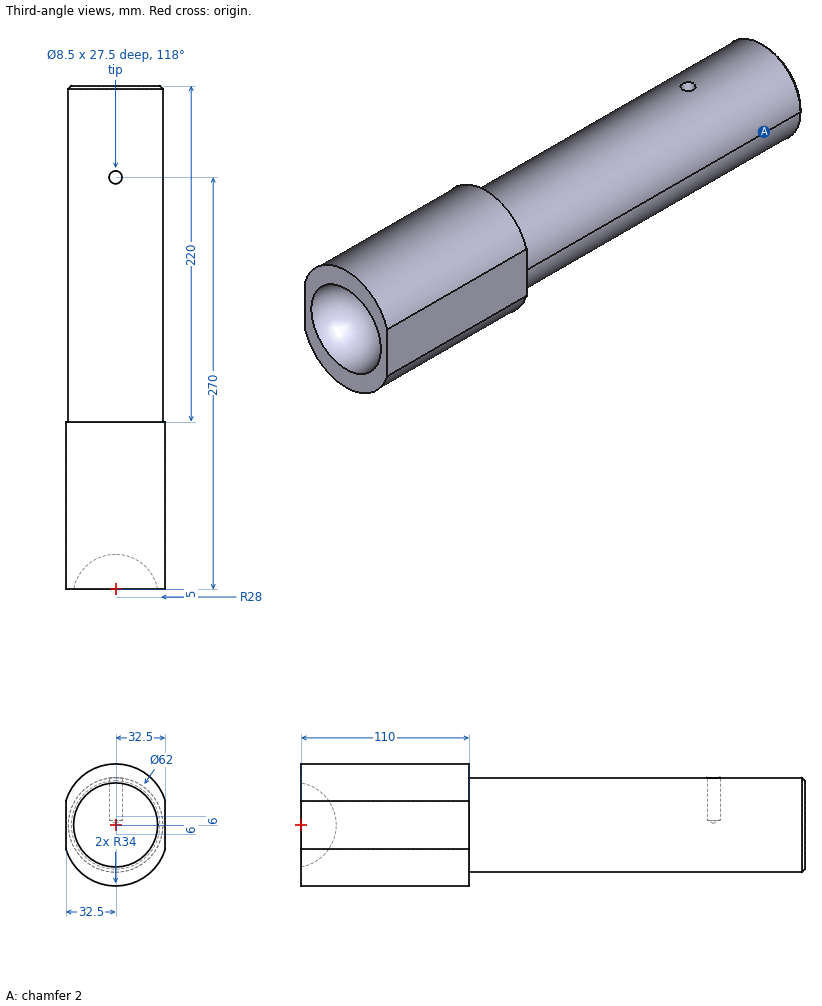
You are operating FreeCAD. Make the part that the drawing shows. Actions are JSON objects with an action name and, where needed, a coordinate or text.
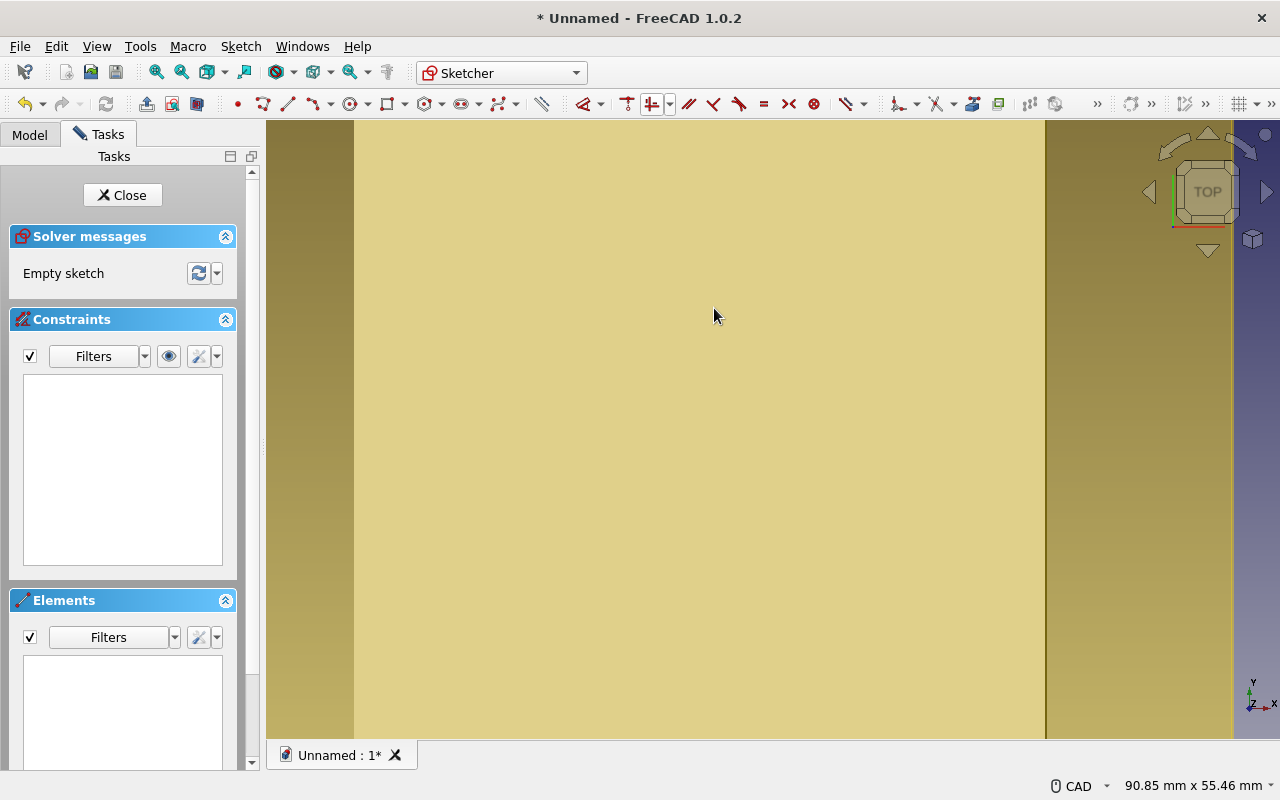
{"action": "scroll", "coordinate": [698, 412], "scroll_direction": "up", "scroll_amount": 7}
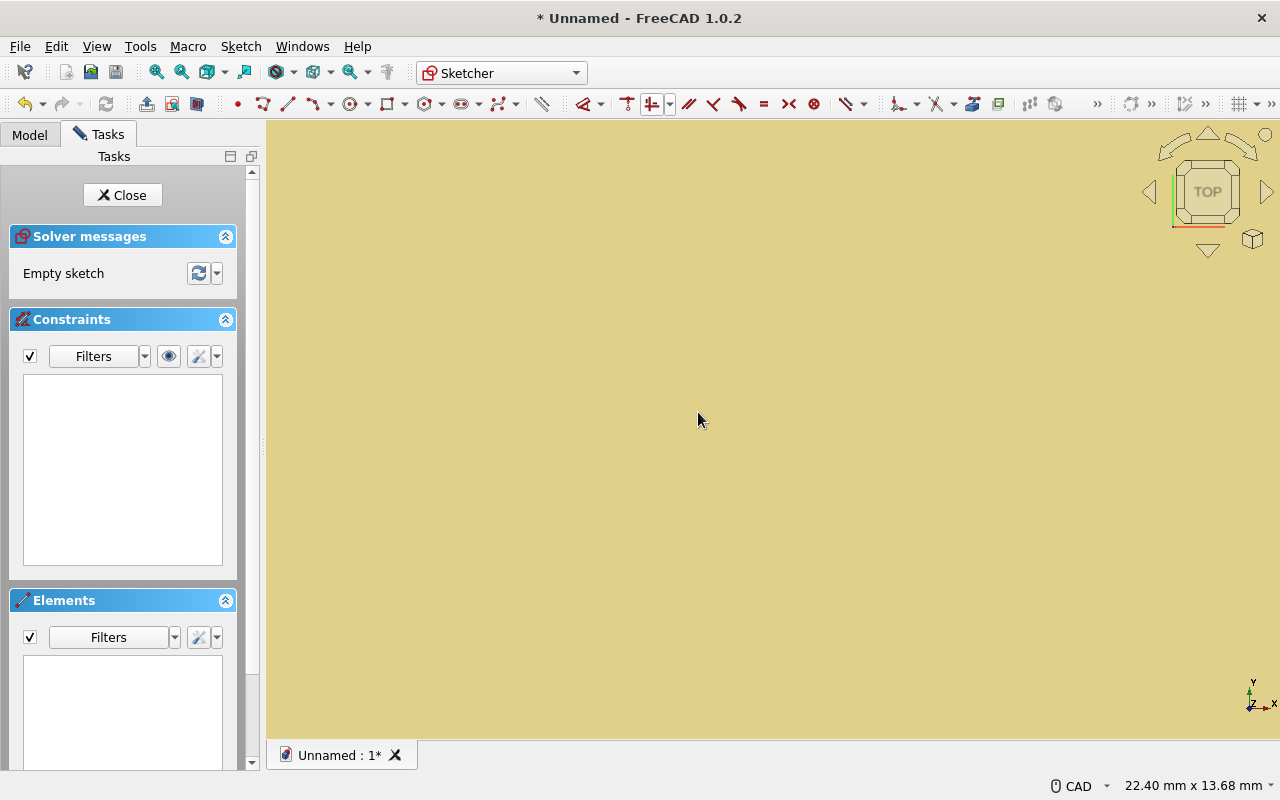
{"action": "key", "text": "g c"}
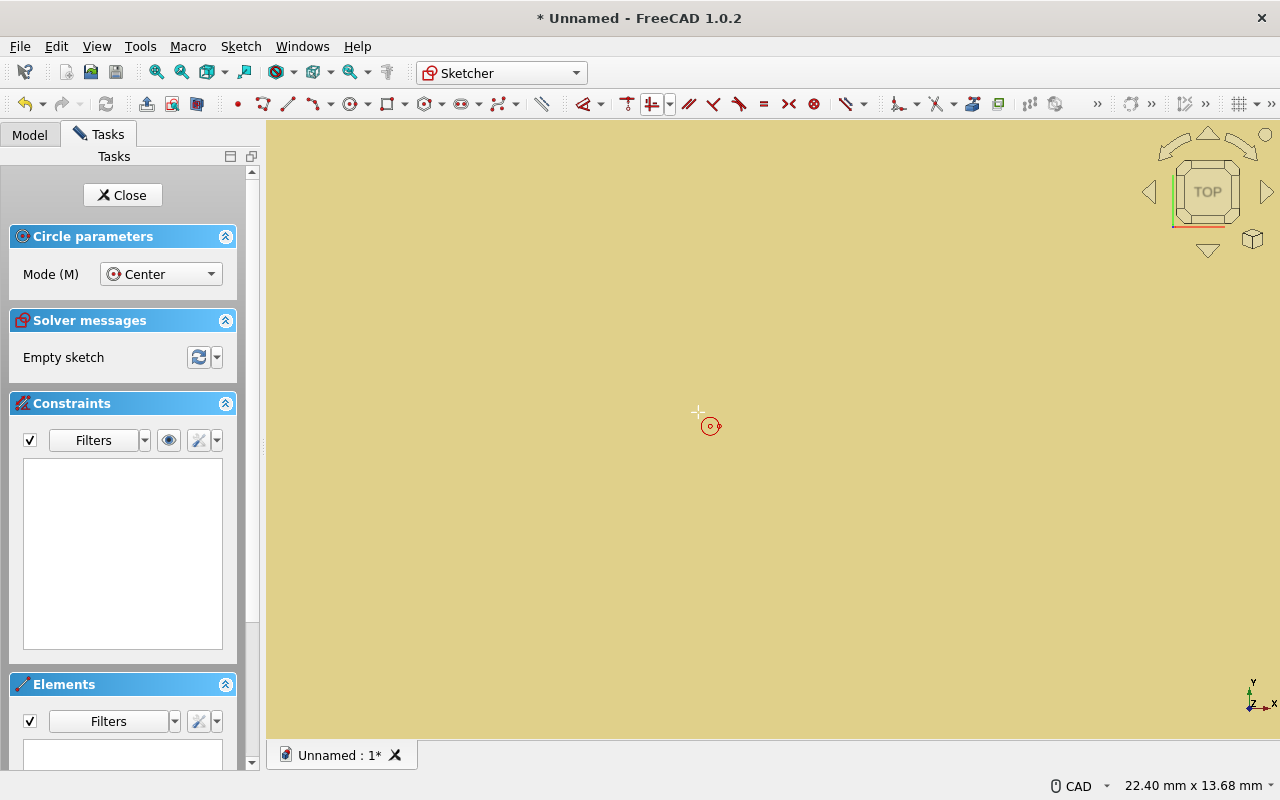
{"action": "left_click", "coordinate": [704, 427]}
{"action": "mouse_move", "coordinate": [840, 291]}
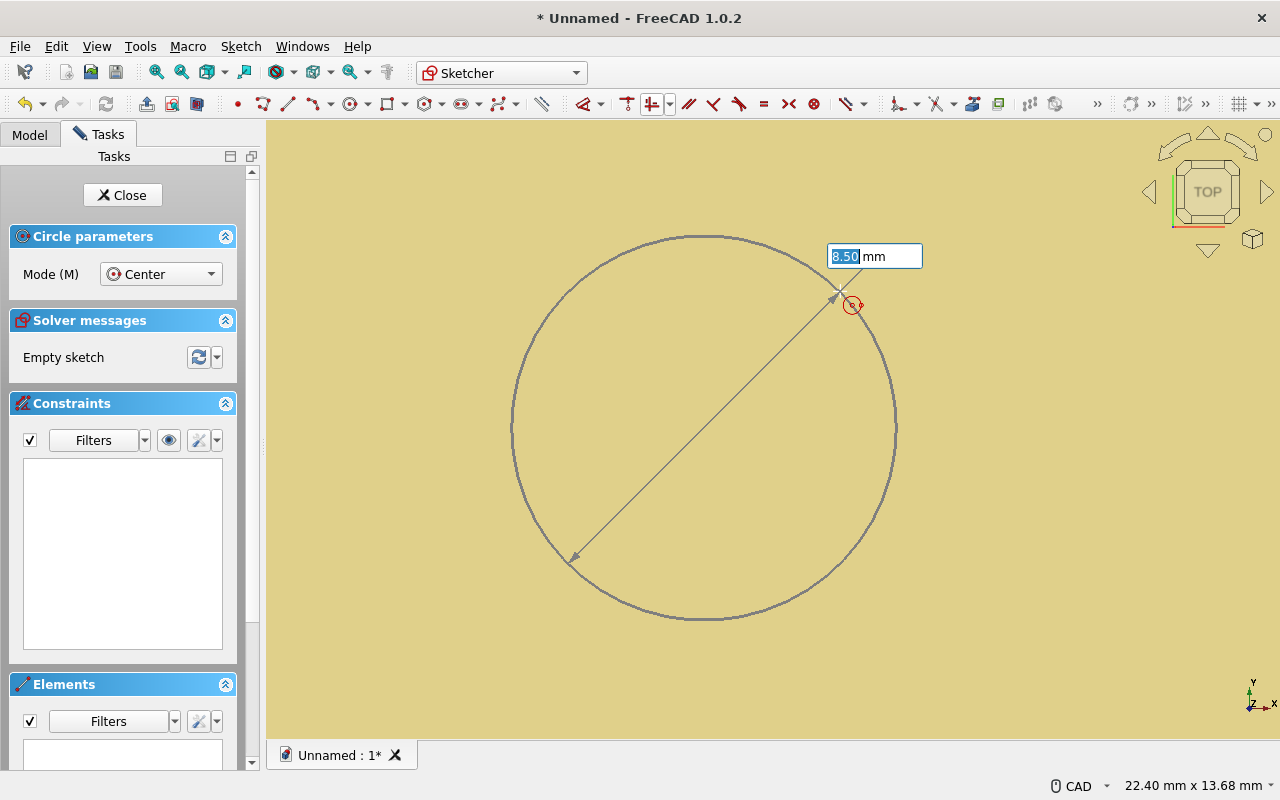
{"action": "type", "text": "8.5"}
{"action": "key", "text": "Return"}
{"action": "key", "text": "Escape"}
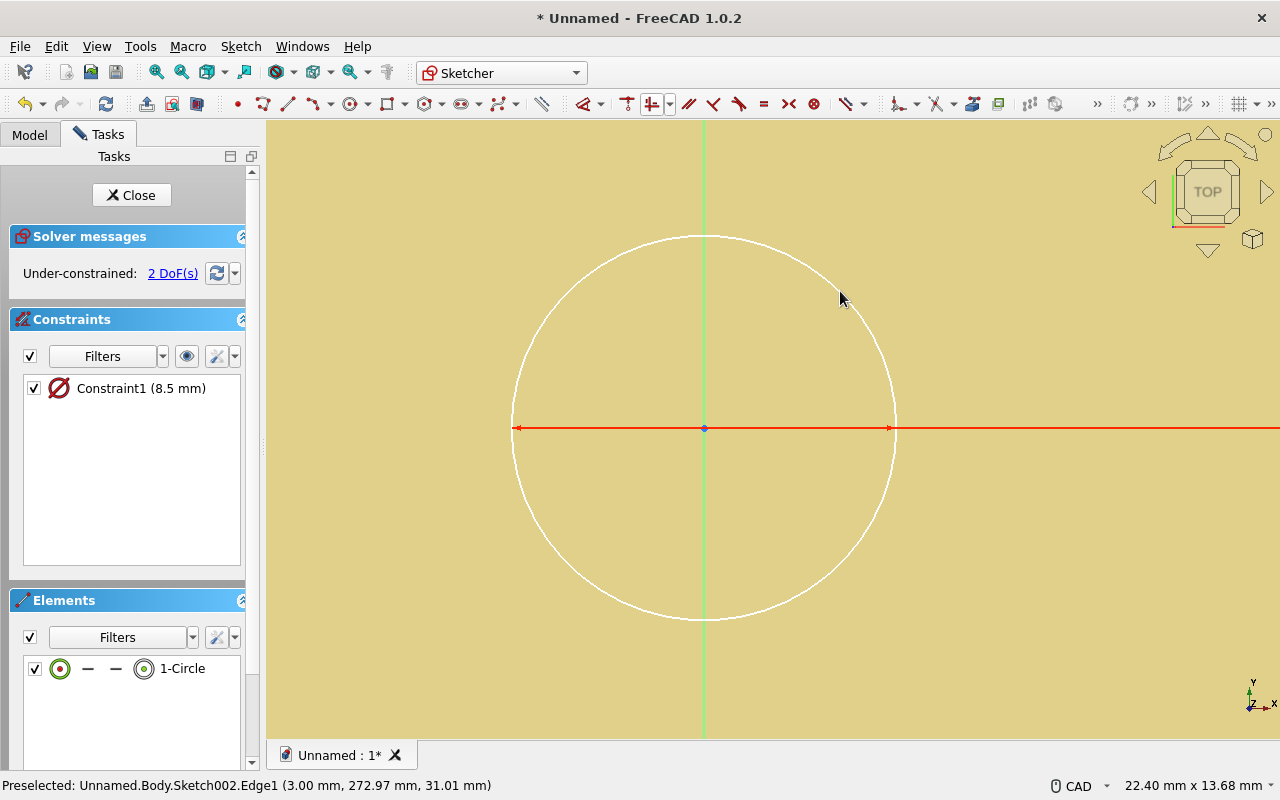
{"action": "left_click", "coordinate": [704, 428]}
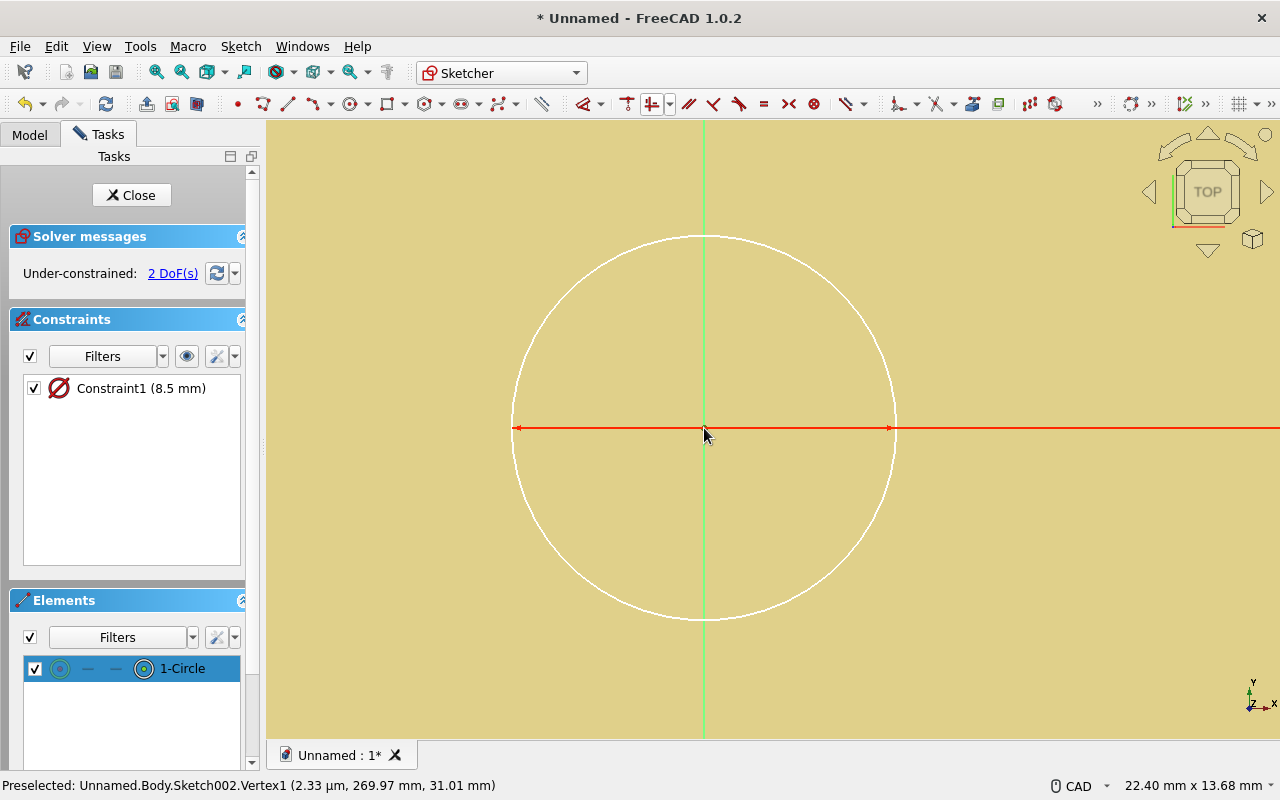
{"action": "left_click", "coordinate": [704, 671]}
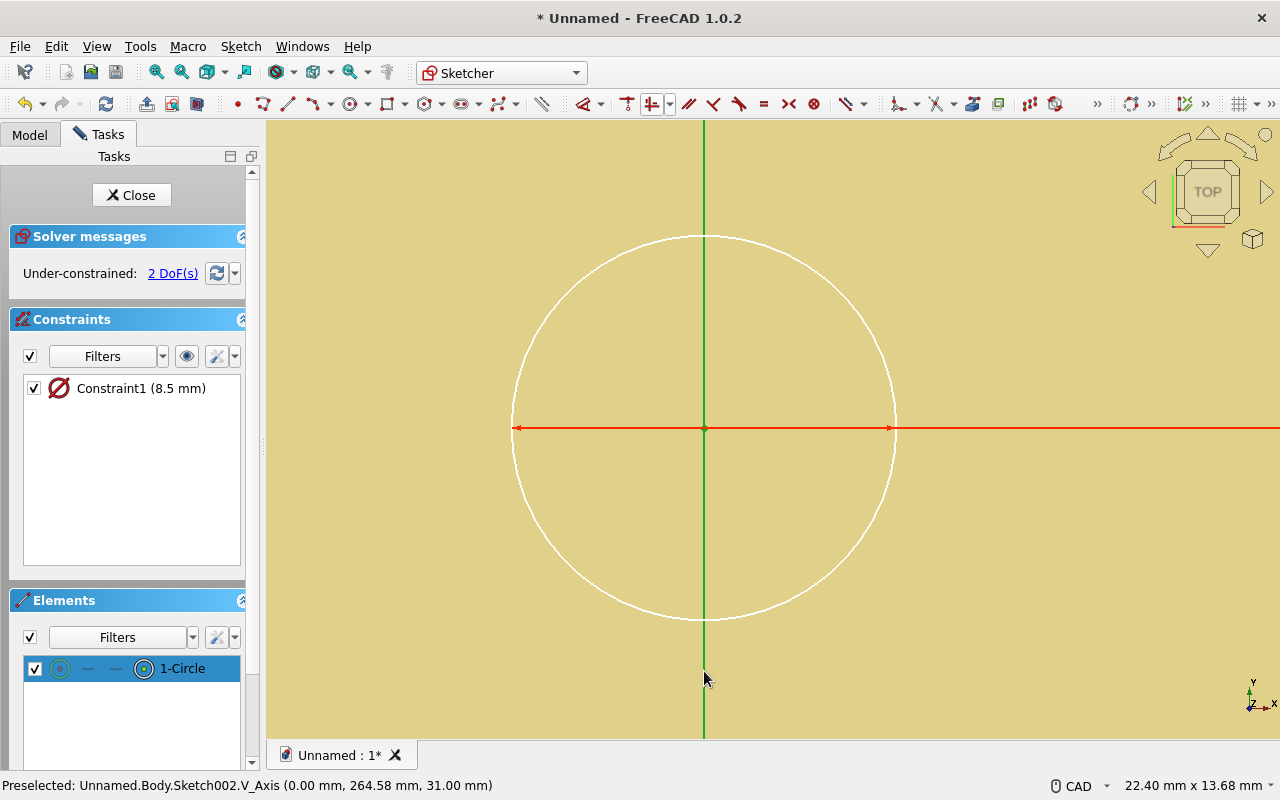
{"action": "left_click", "coordinate": [627, 104]}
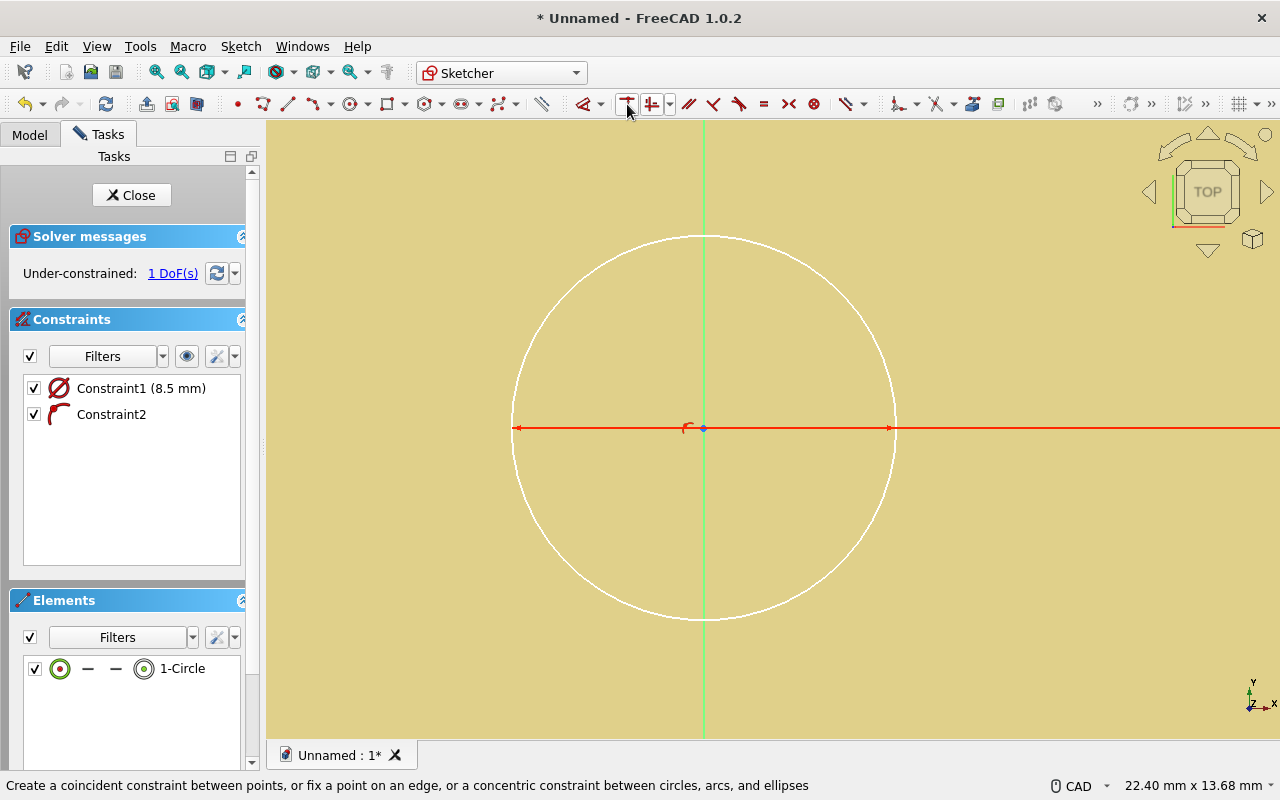
{"action": "key", "text": "d"}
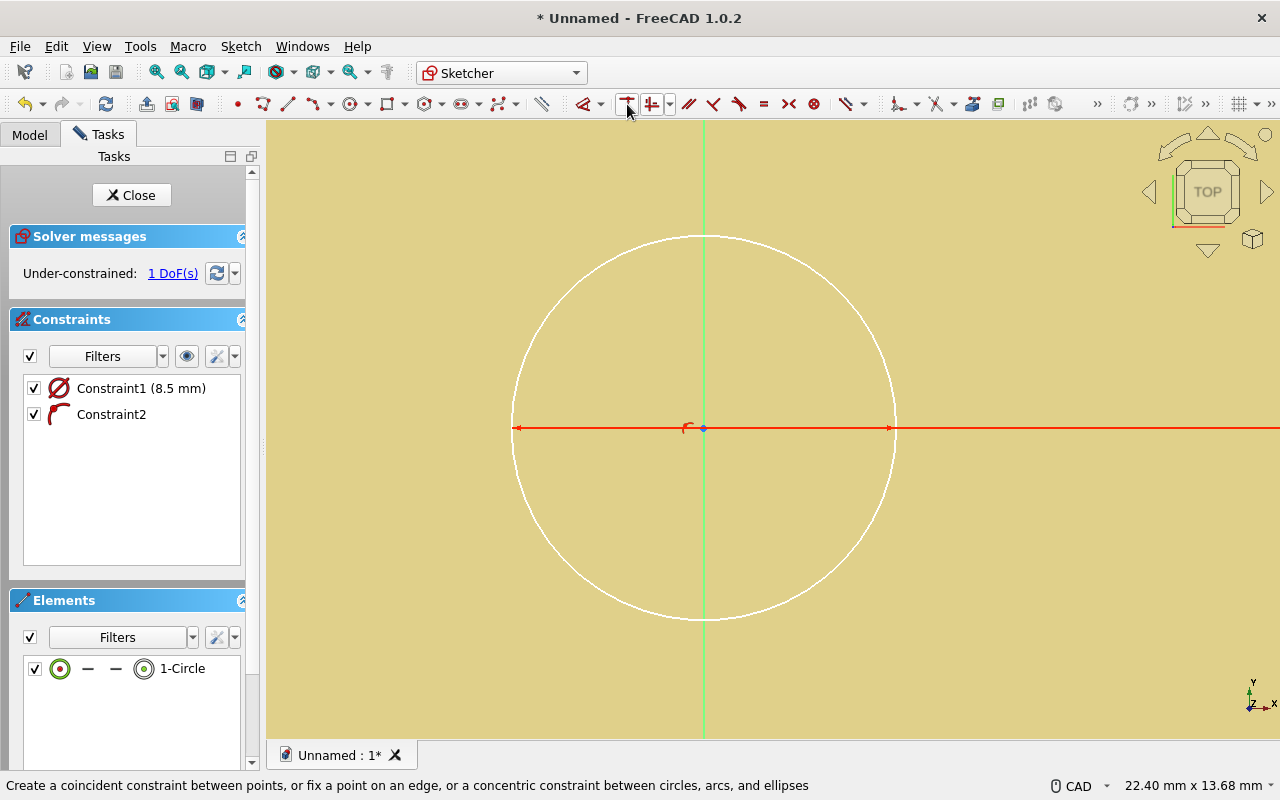
{"action": "left_click", "coordinate": [704, 428]}
{"action": "left_click", "coordinate": [738, 569]}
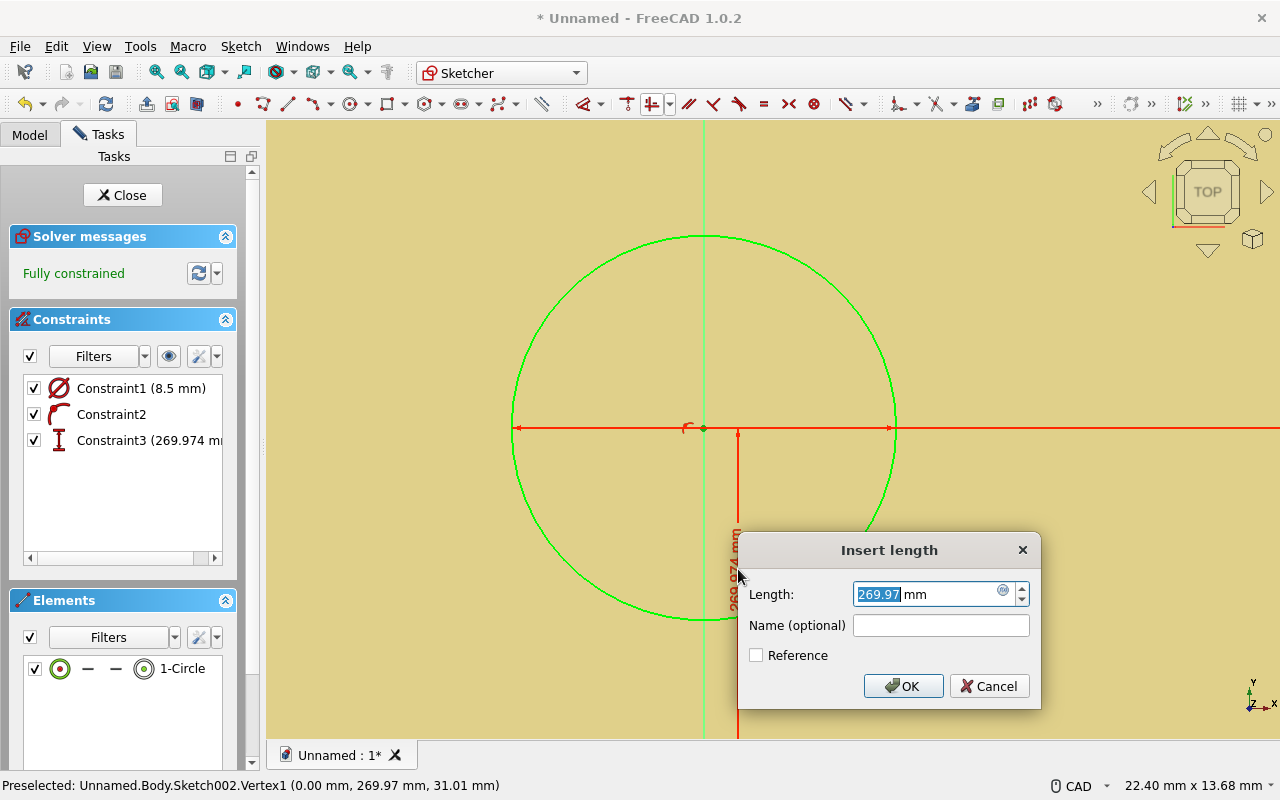
{"action": "type", "text": "270"}
{"action": "key", "text": "Return"}
{"action": "key", "text": "Escape"}